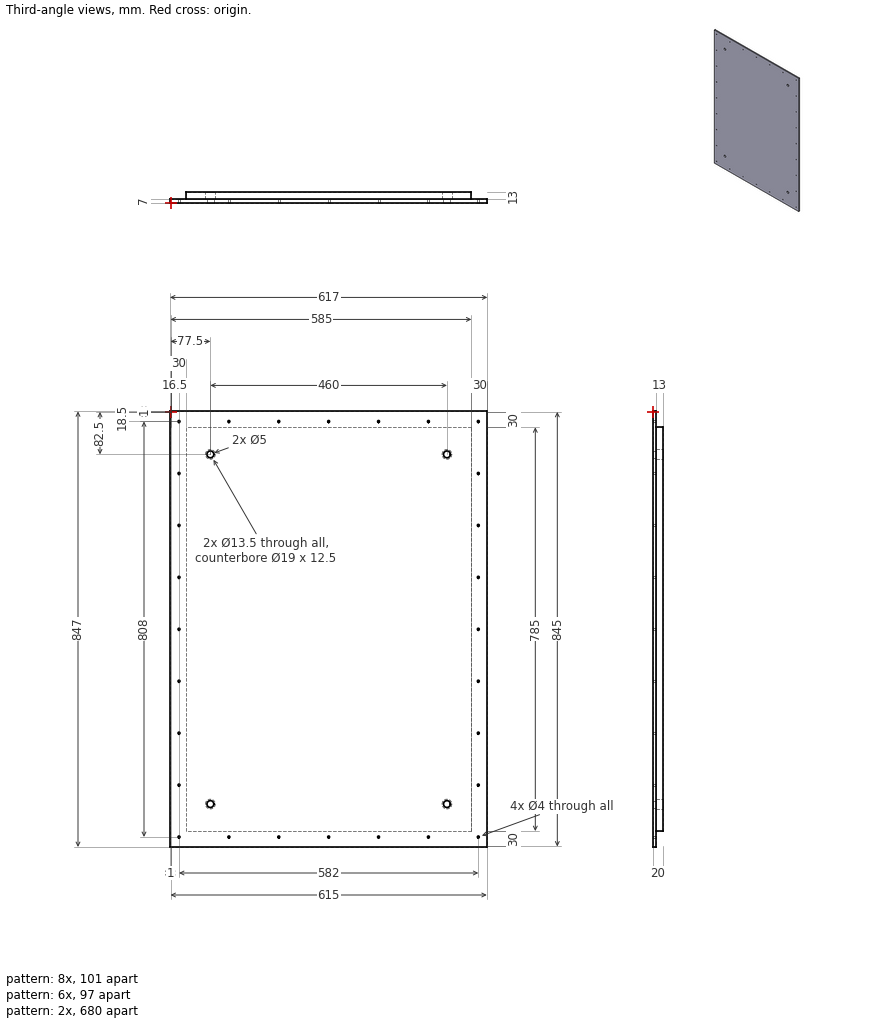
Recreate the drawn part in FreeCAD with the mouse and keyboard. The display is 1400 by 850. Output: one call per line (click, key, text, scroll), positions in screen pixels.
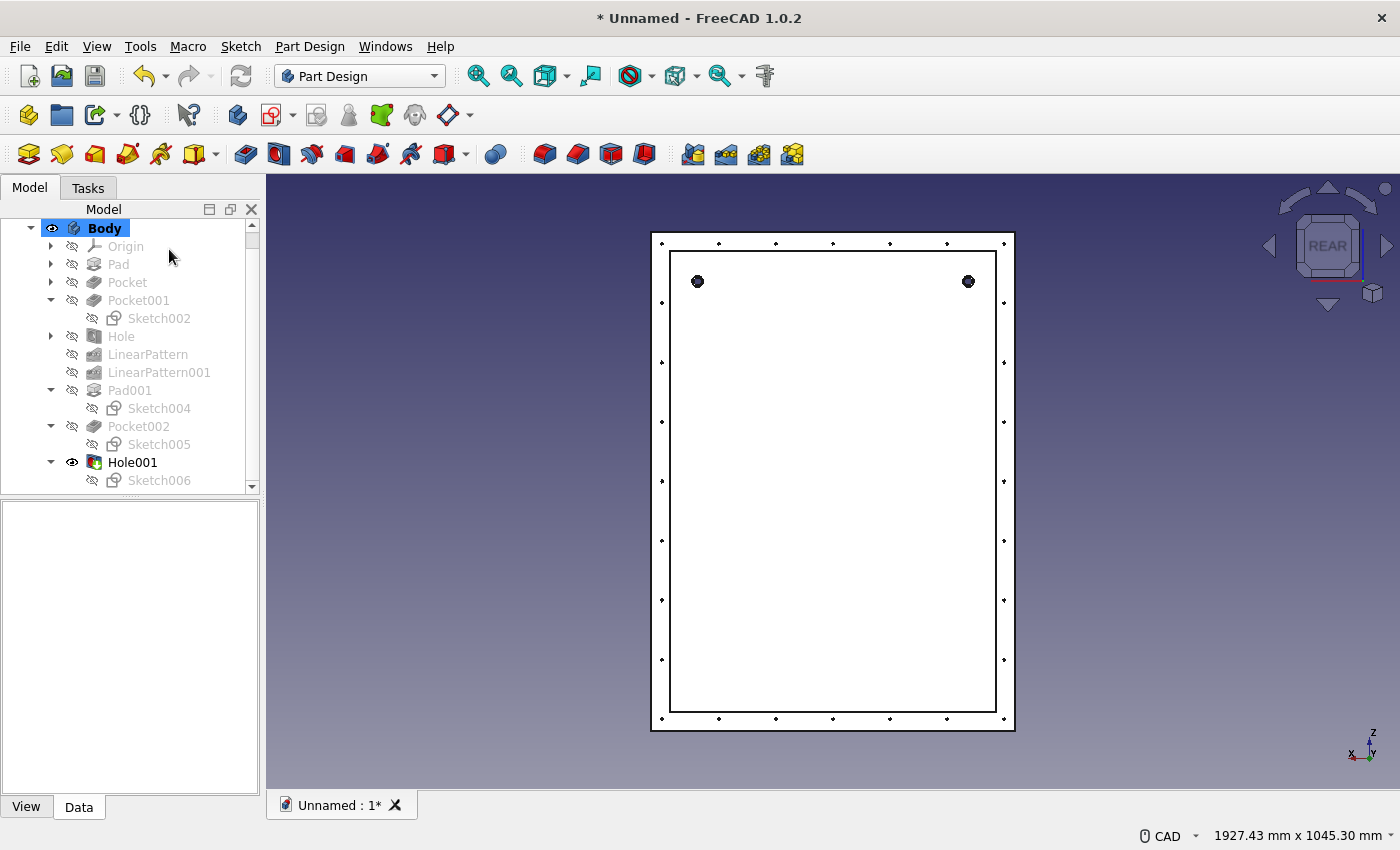
click(117, 462)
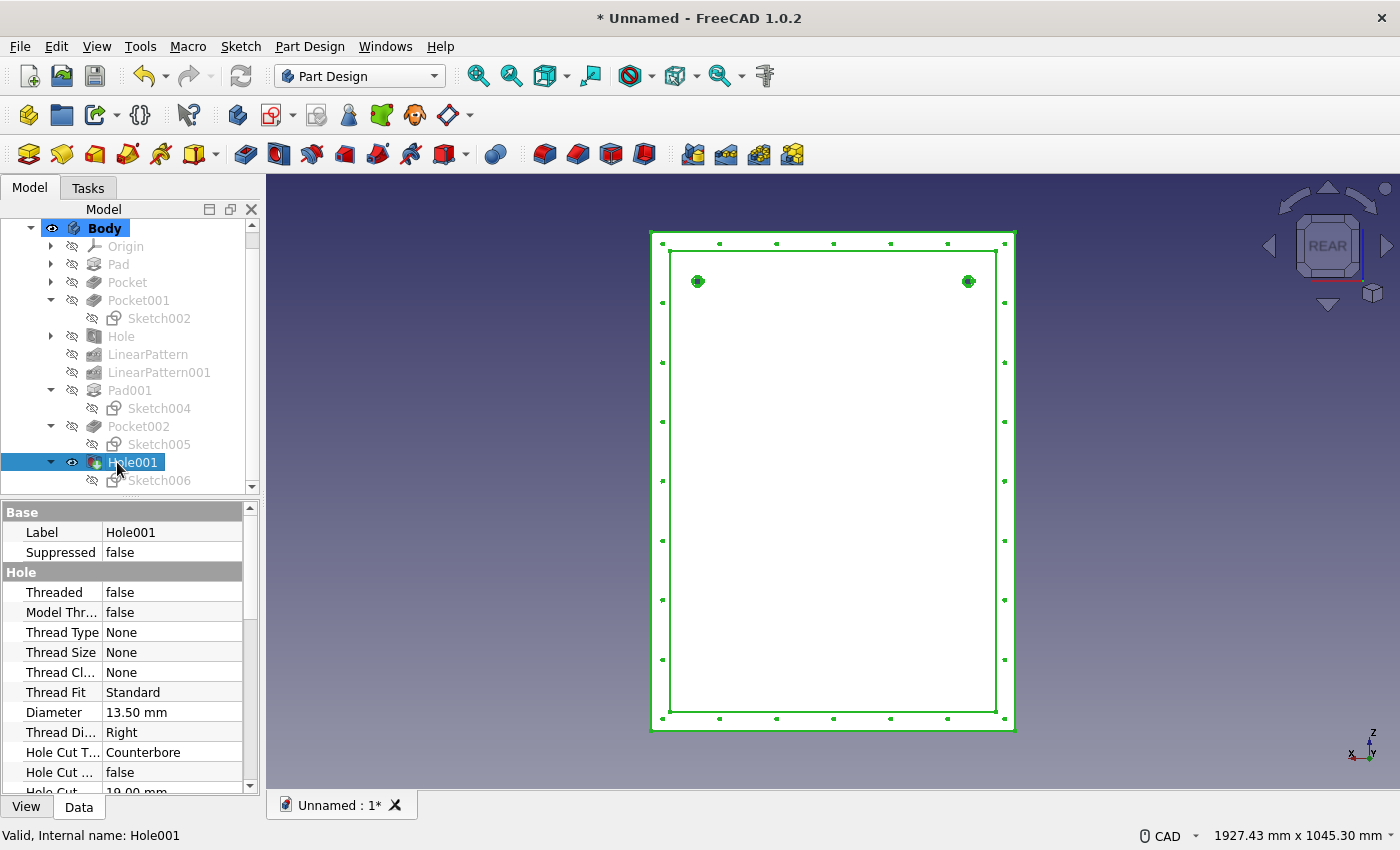
click(726, 154)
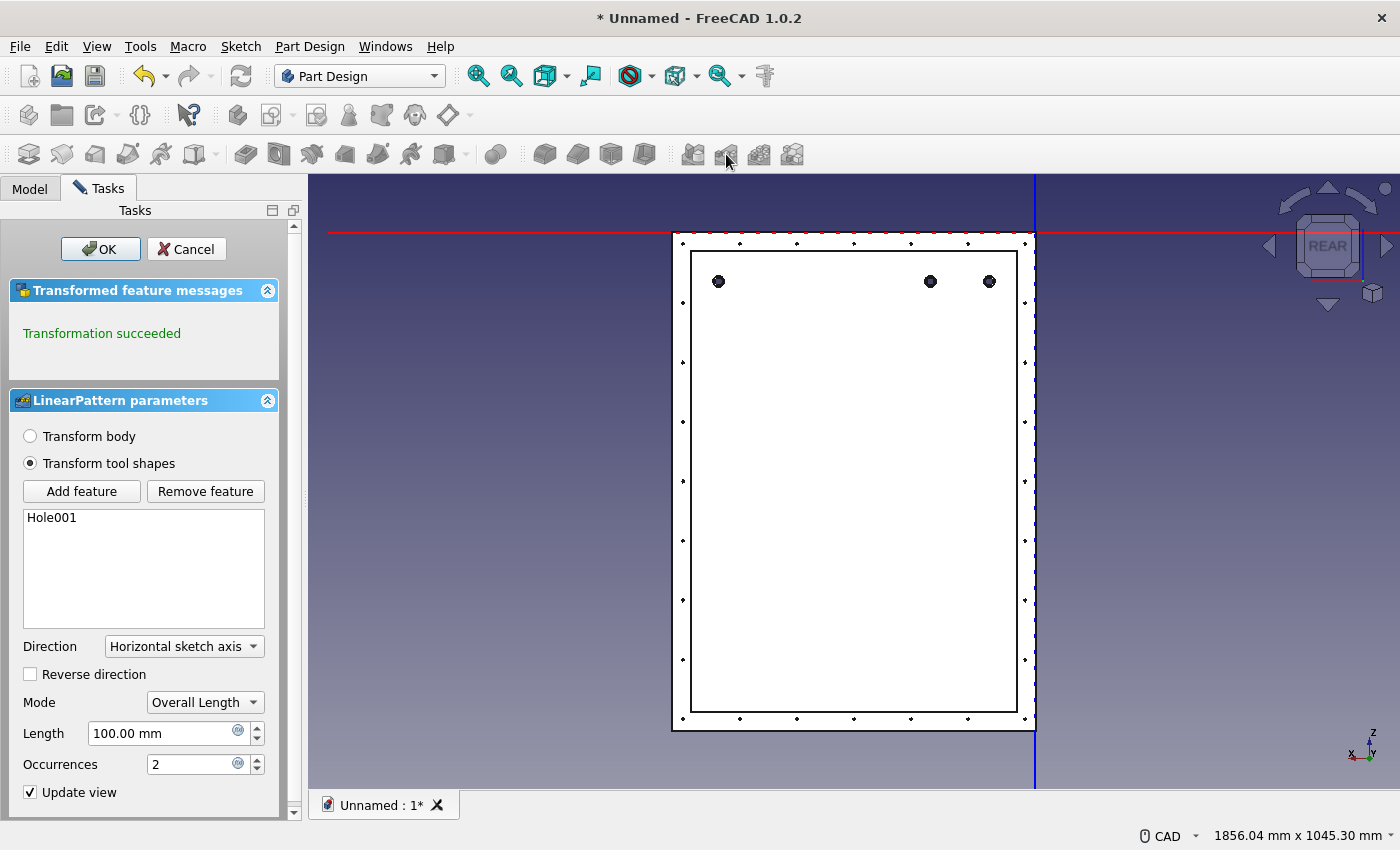
click(185, 646)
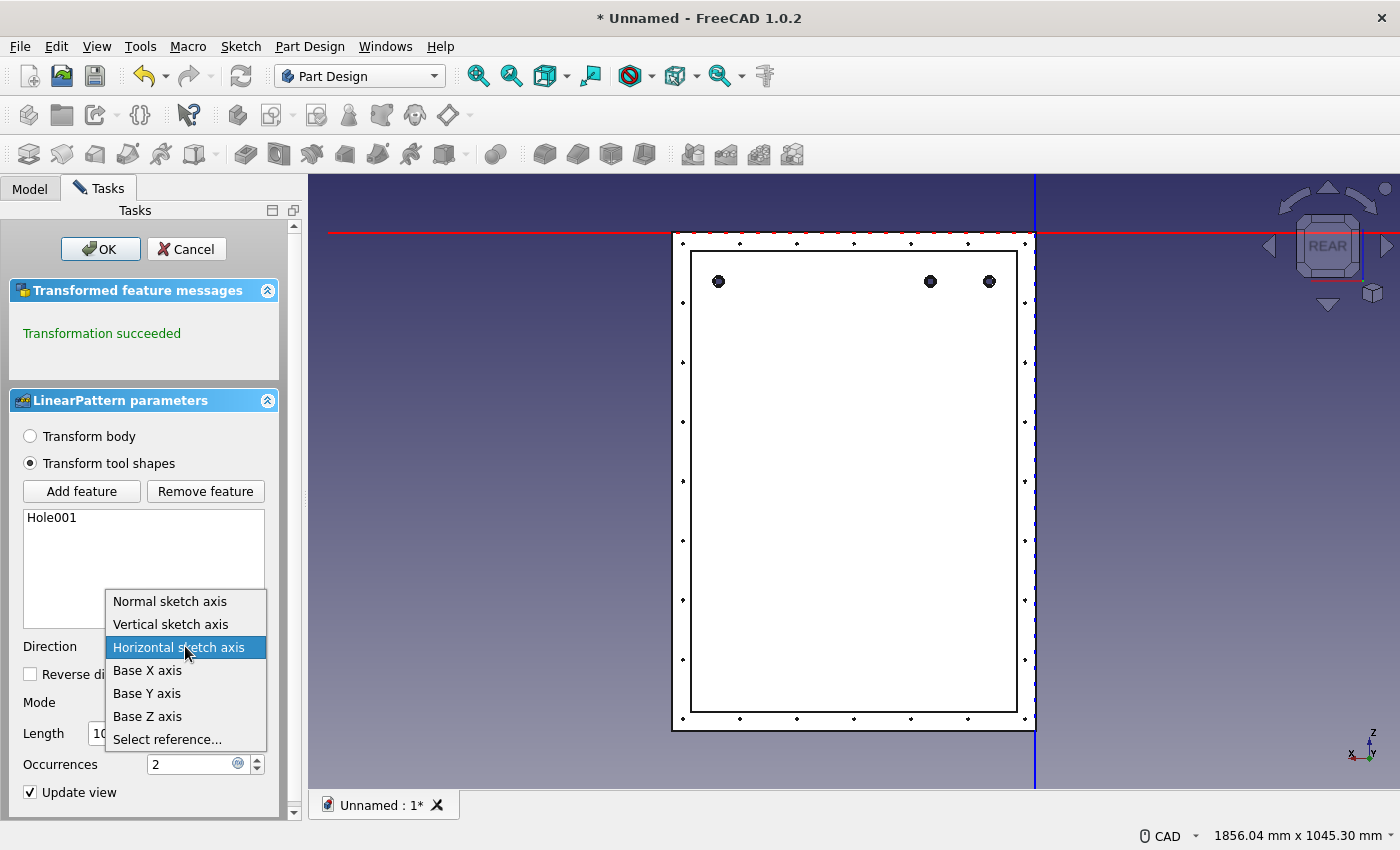
click(184, 716)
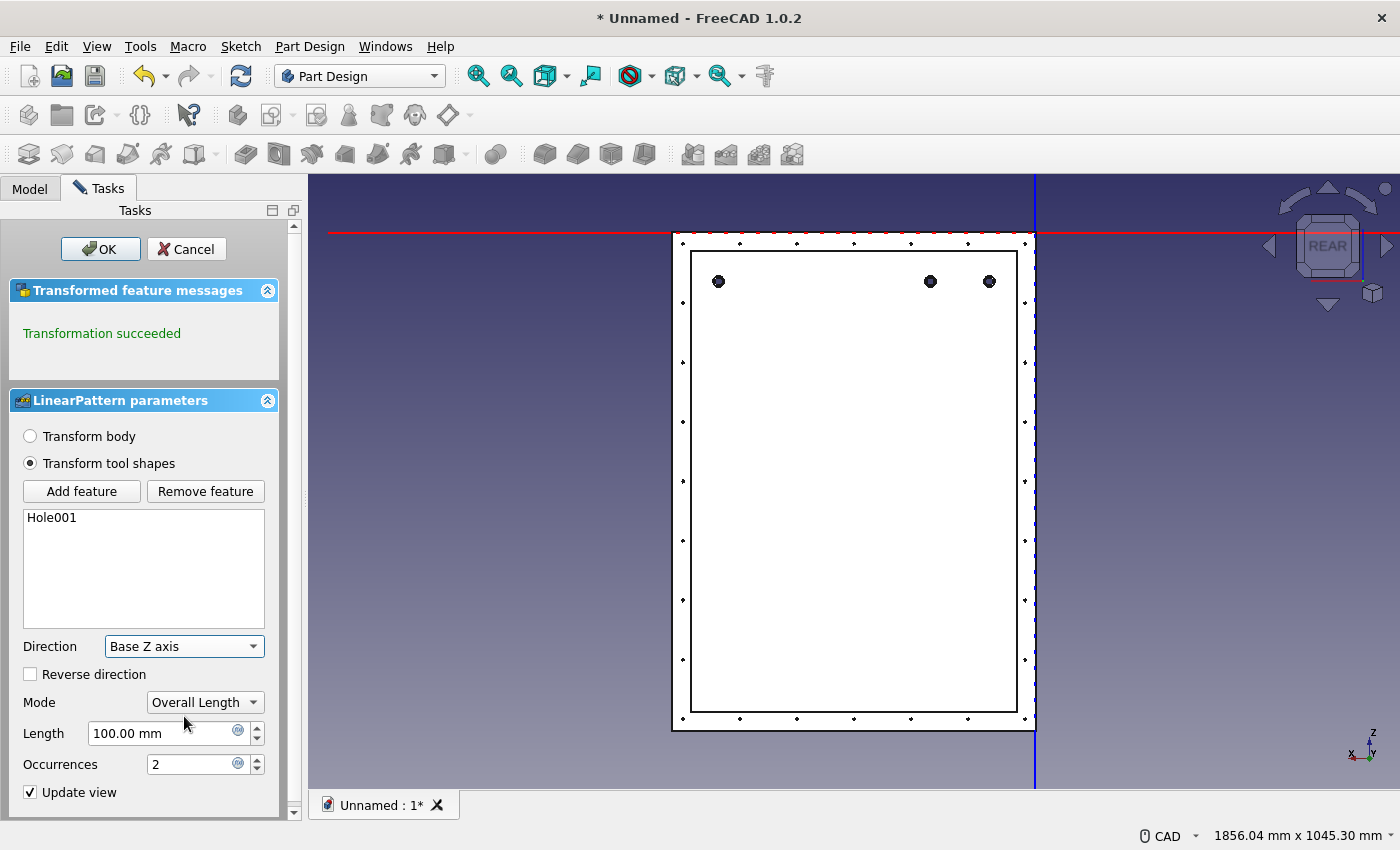
click(206, 702)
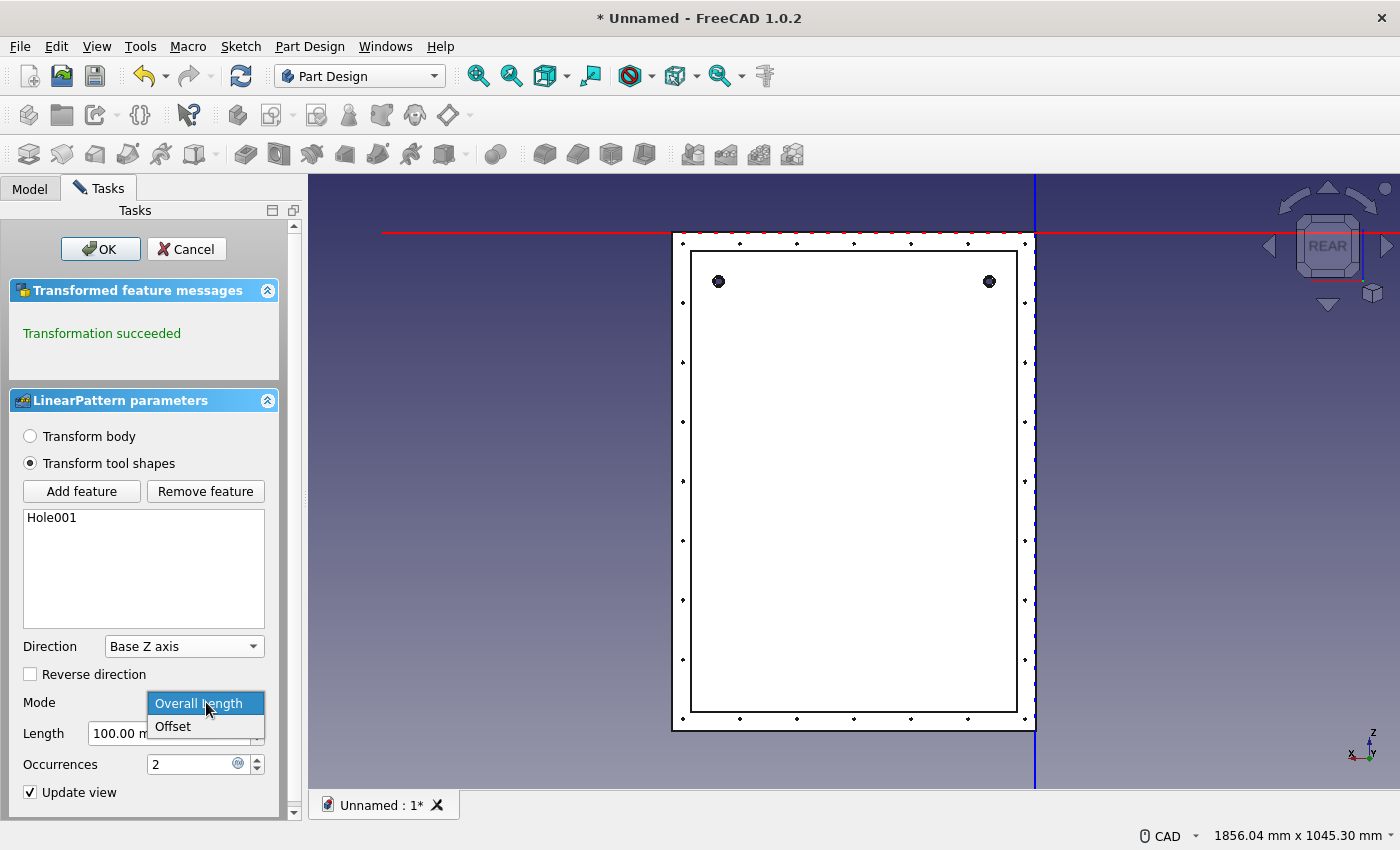
click(204, 726)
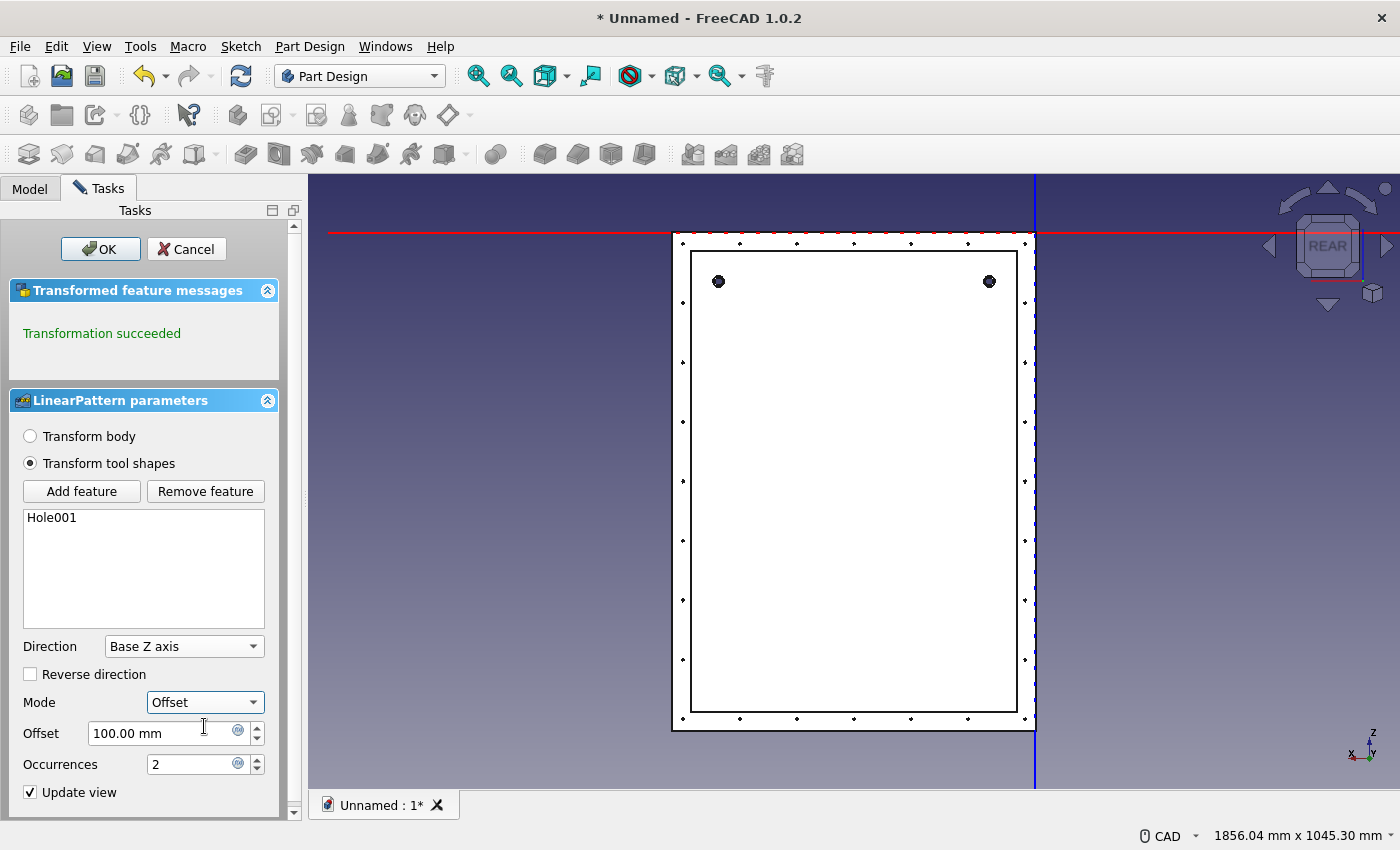
triple_click(170, 734)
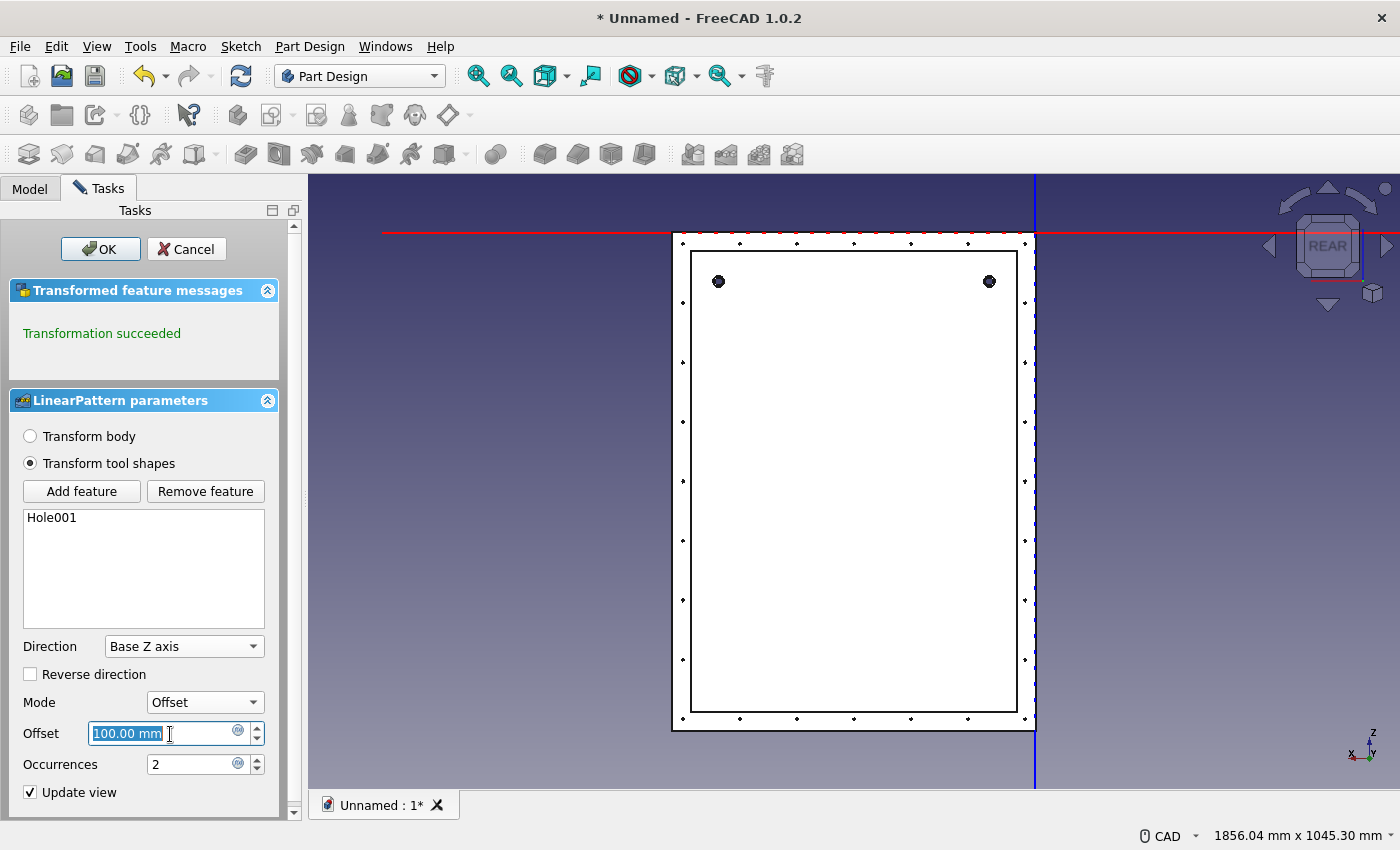
text(680)
key(Tab)